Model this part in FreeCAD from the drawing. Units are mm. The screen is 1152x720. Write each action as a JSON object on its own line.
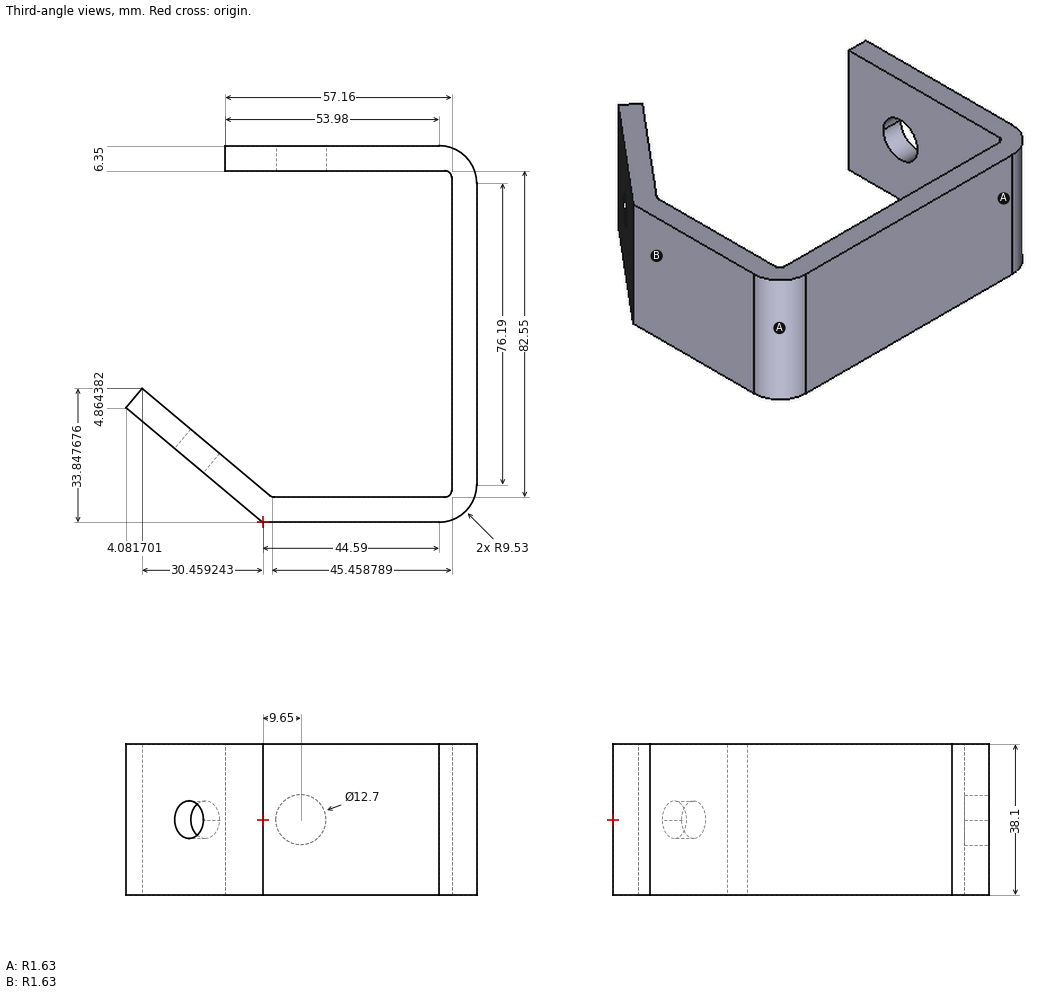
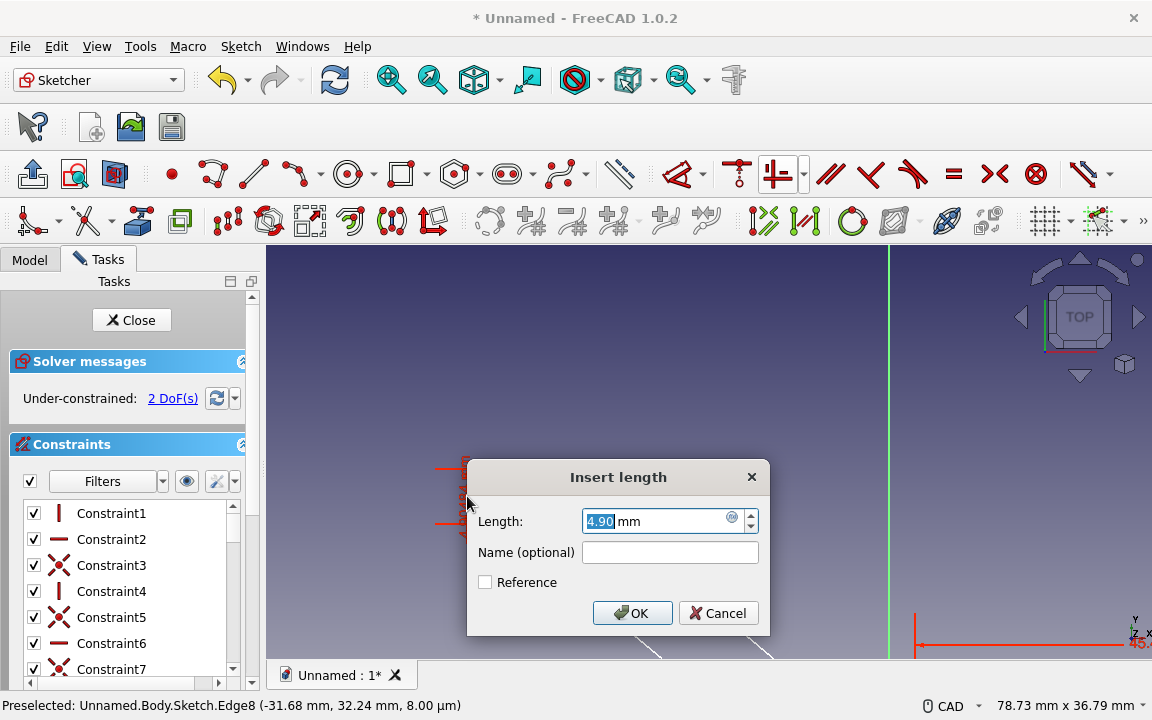
{"action": "type", "text": "4.864382"}
{"action": "key", "text": "Return"}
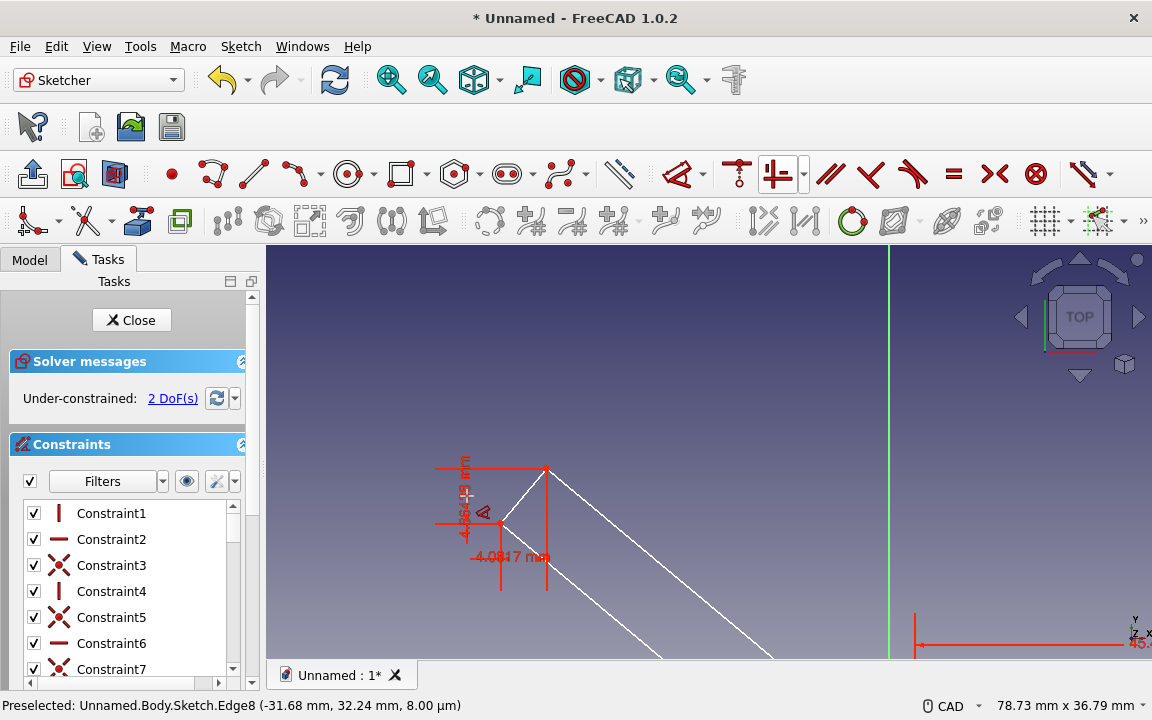
{"action": "scroll", "coordinate": [523, 498], "scroll_direction": "down", "scroll_amount": 7}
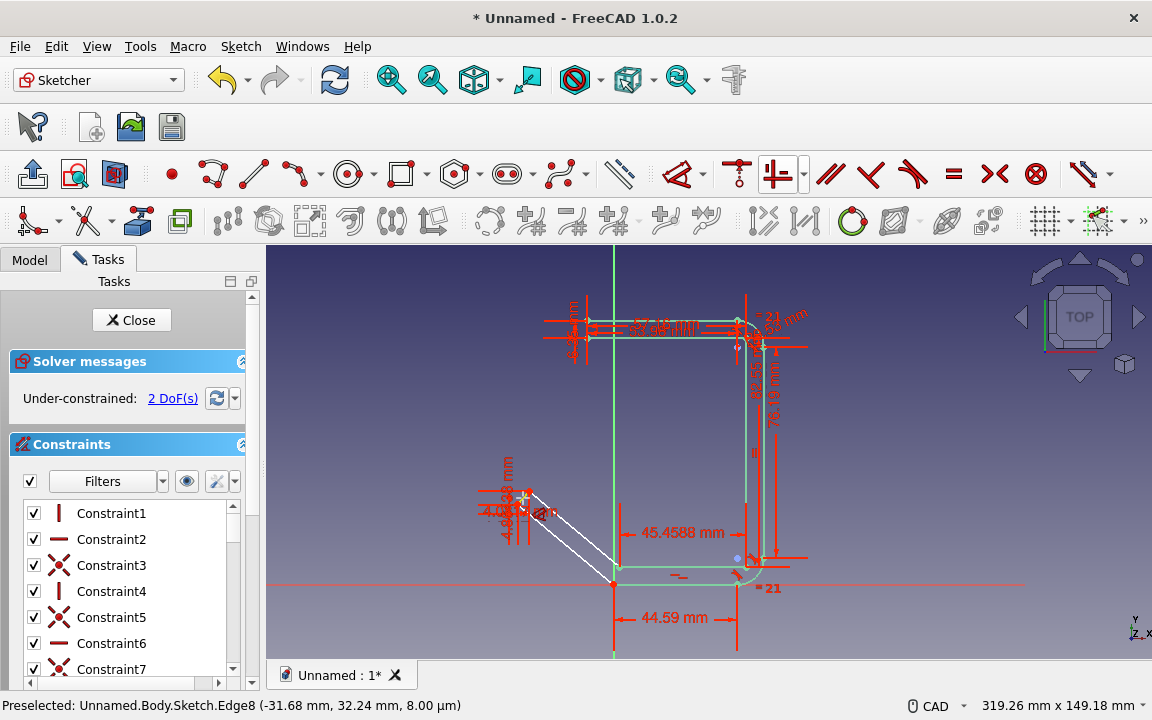
{"action": "left_click", "coordinate": [529, 491]}
{"action": "left_click", "coordinate": [571, 619]}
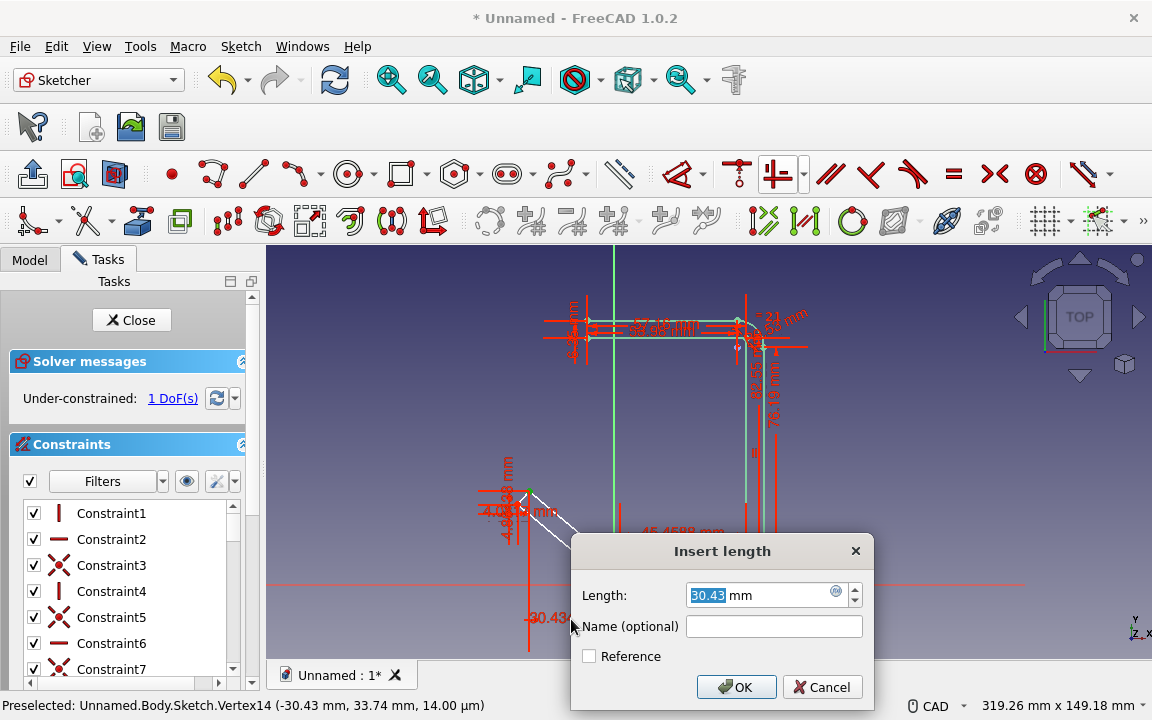
{"action": "type", "text": "30.459243"}
{"action": "key", "text": "Return"}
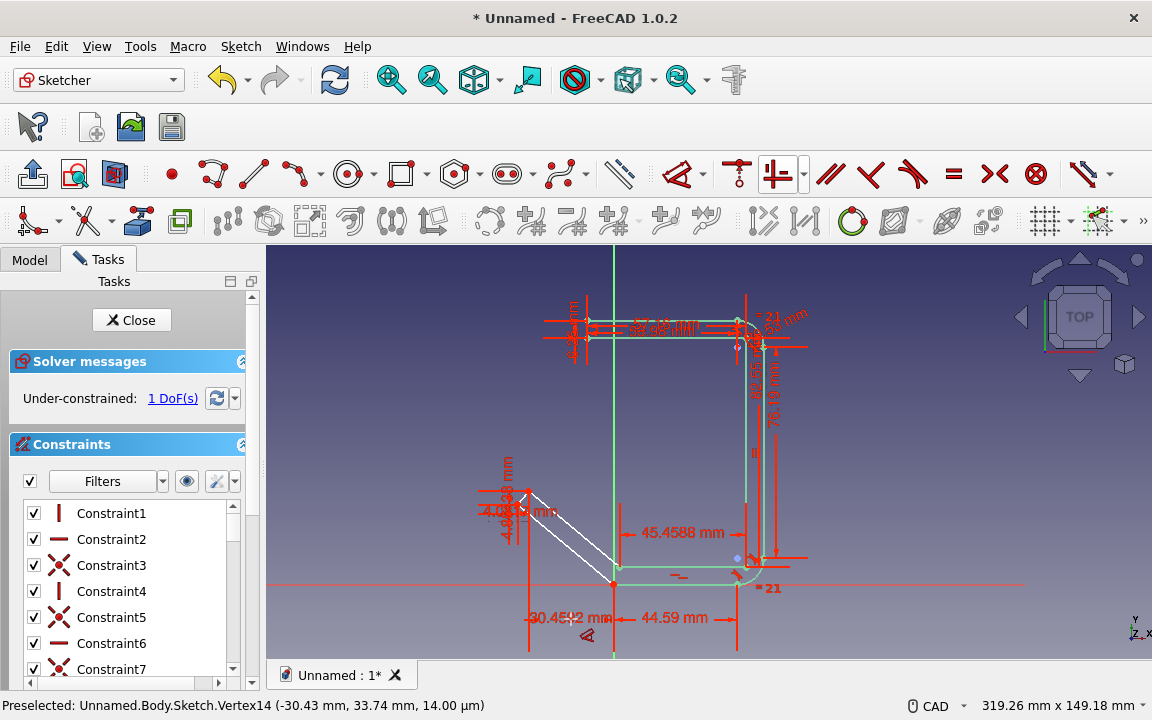
{"action": "left_click", "coordinate": [529, 491]}
{"action": "left_click", "coordinate": [495, 538]}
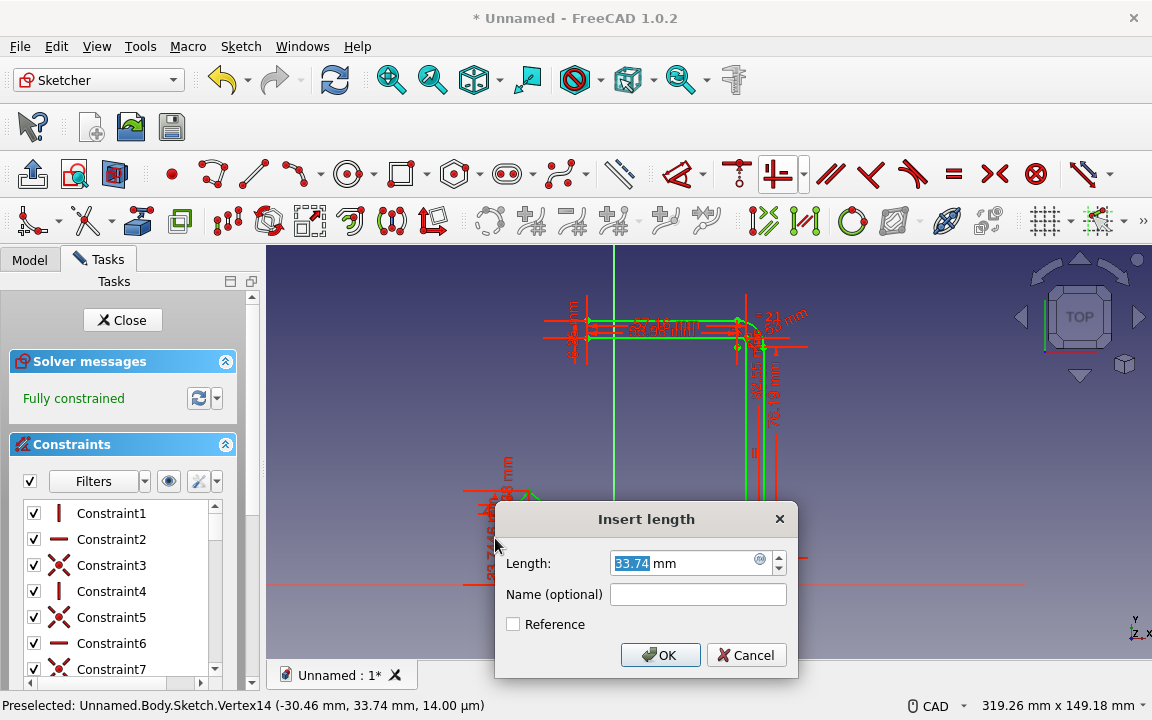
{"action": "type", "text": "33.847676"}
{"action": "key", "text": "Return"}
{"action": "key", "text": "Escape"}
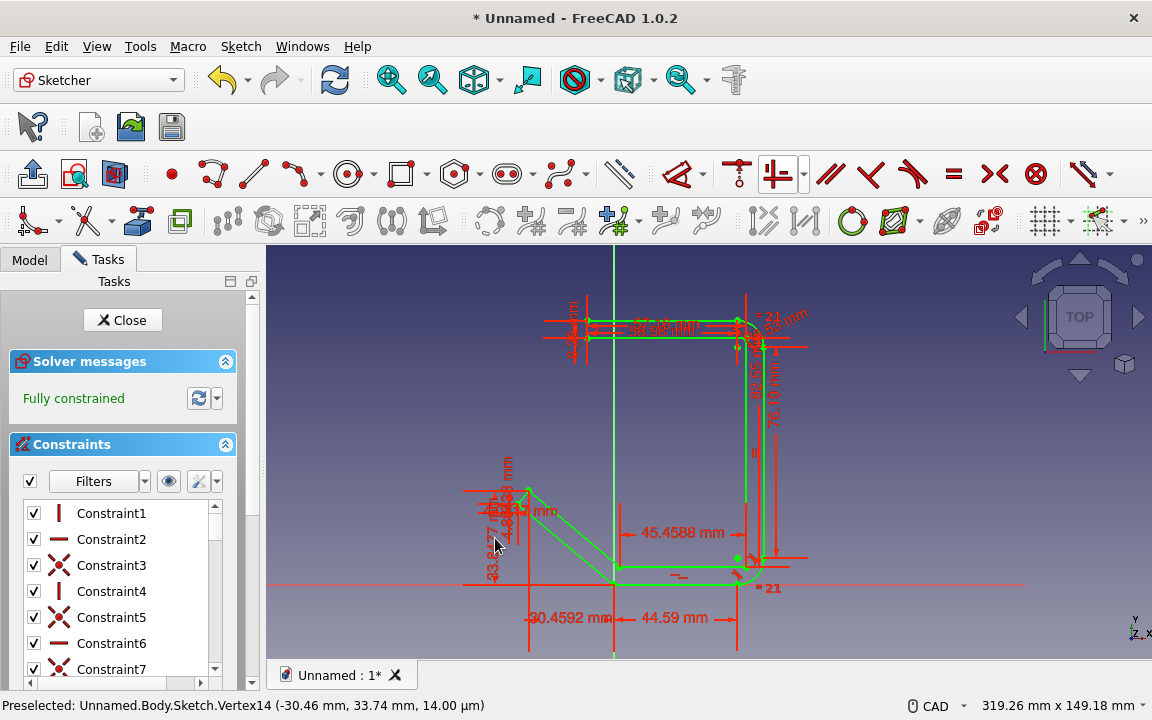
{"action": "left_click", "coordinate": [123, 320]}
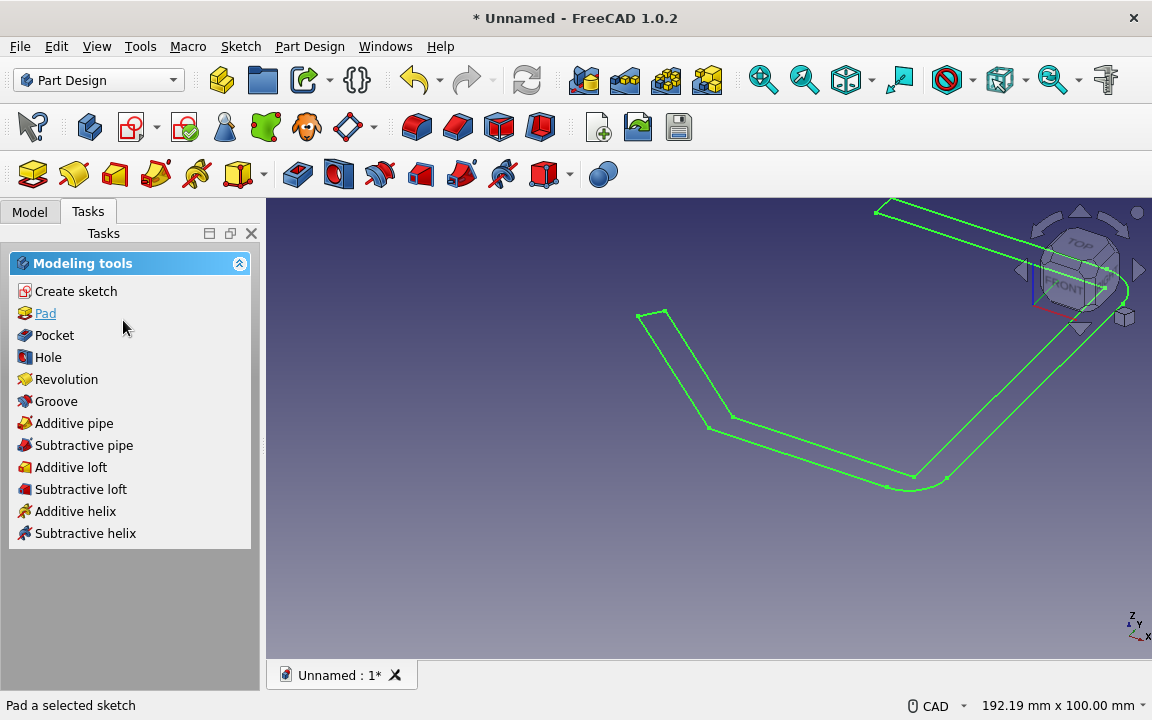
{"action": "left_click", "coordinate": [33, 174]}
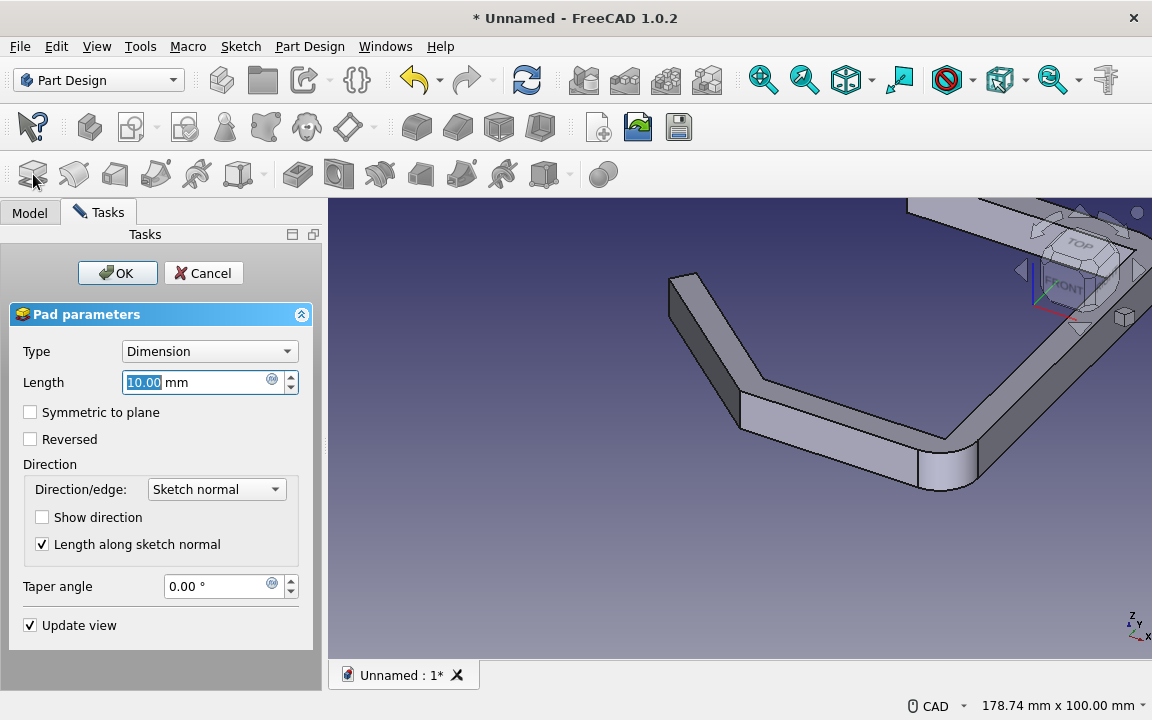
{"action": "type", "text": "38.1"}
{"action": "key", "text": "Tab"}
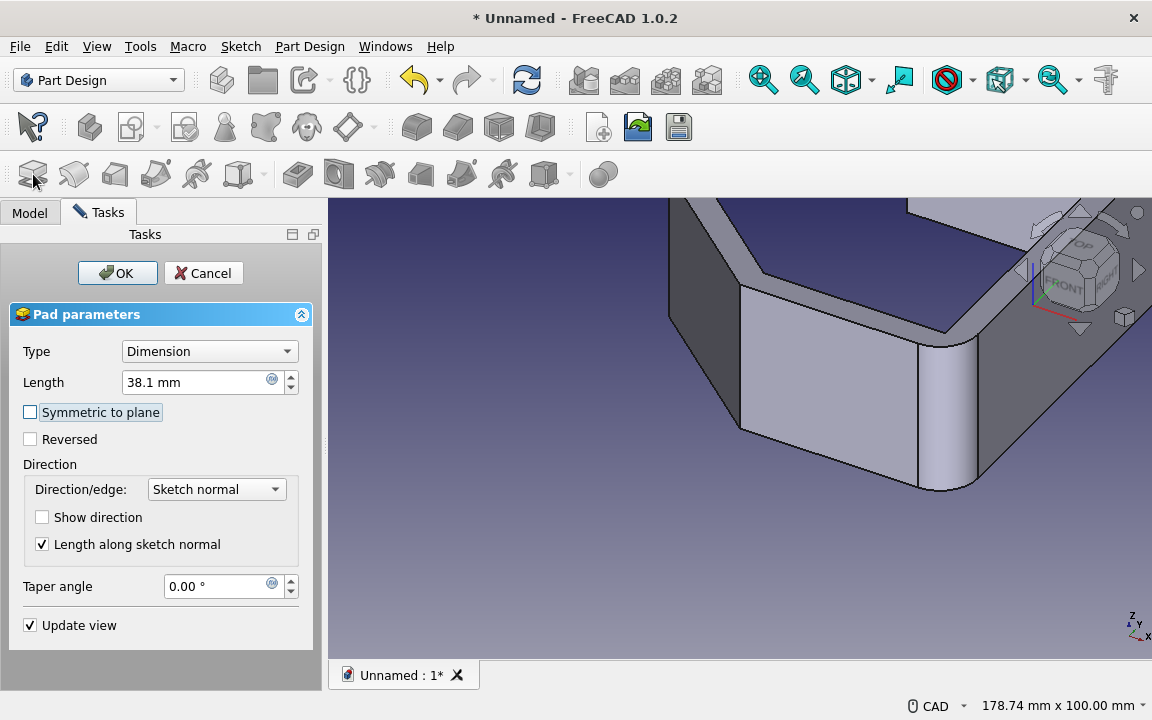
{"action": "left_click", "coordinate": [31, 412]}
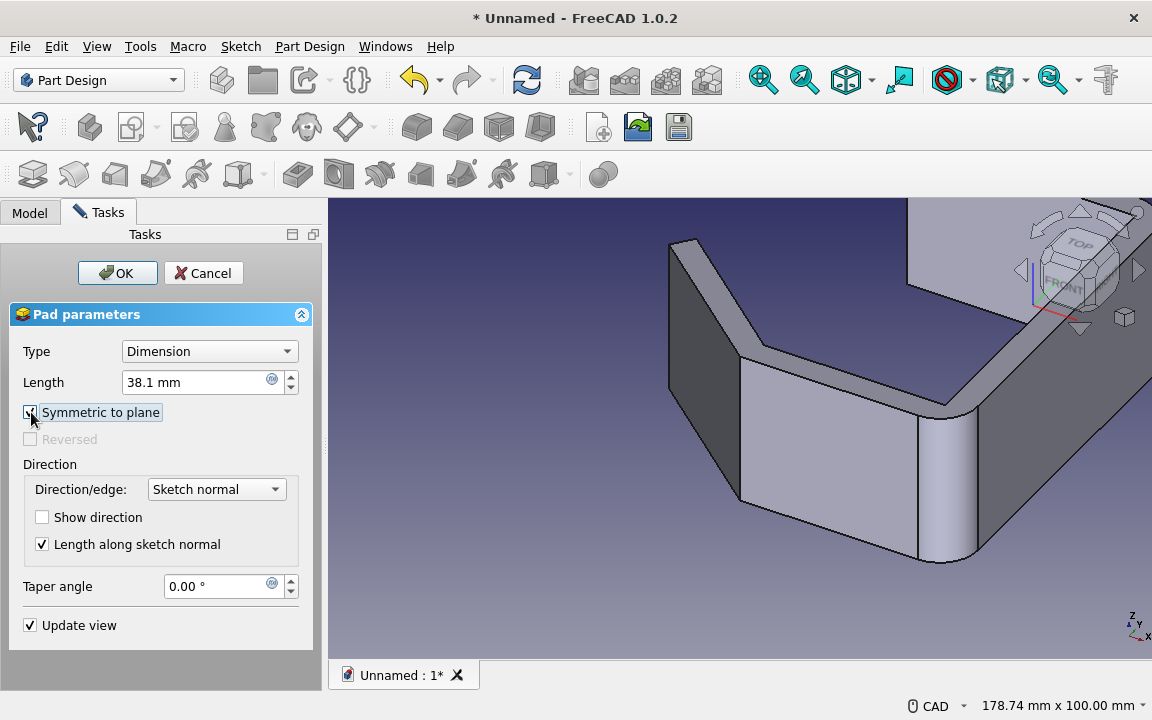
{"action": "left_click", "coordinate": [118, 273]}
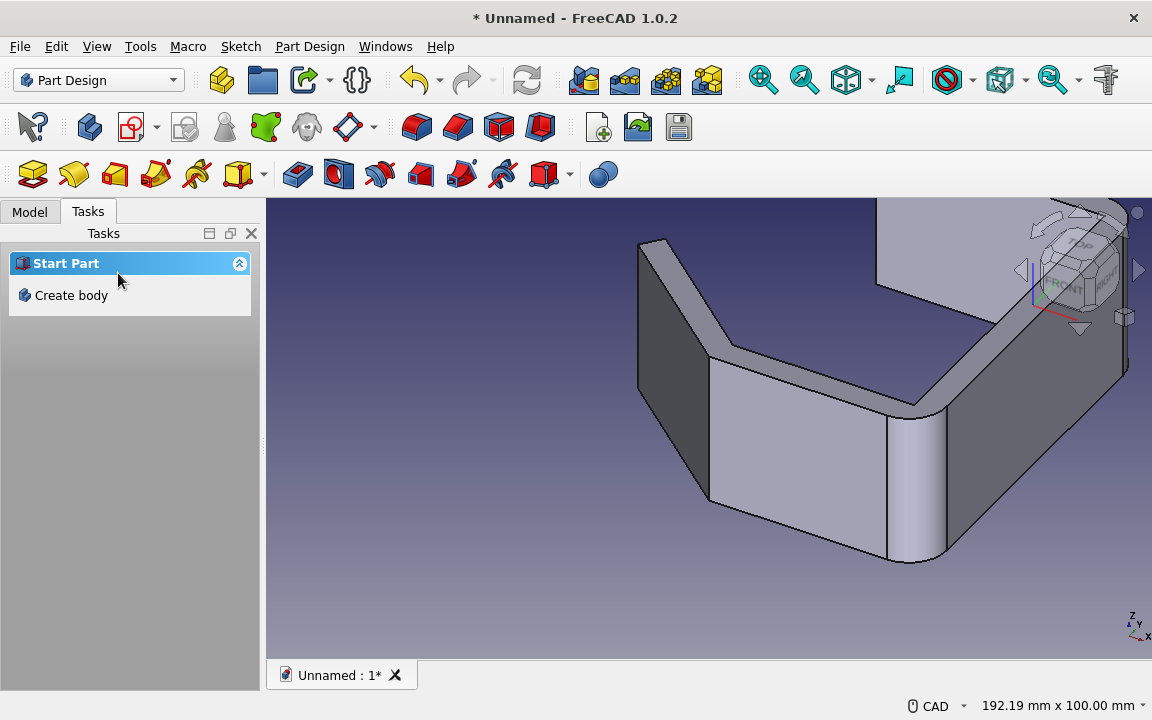
{"action": "key", "text": "v f"}